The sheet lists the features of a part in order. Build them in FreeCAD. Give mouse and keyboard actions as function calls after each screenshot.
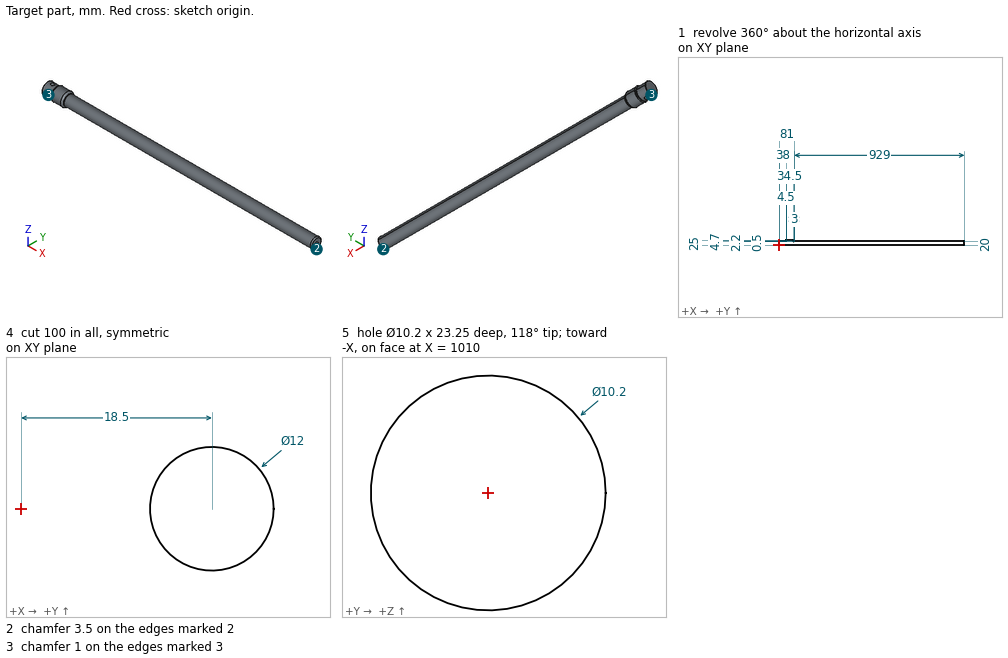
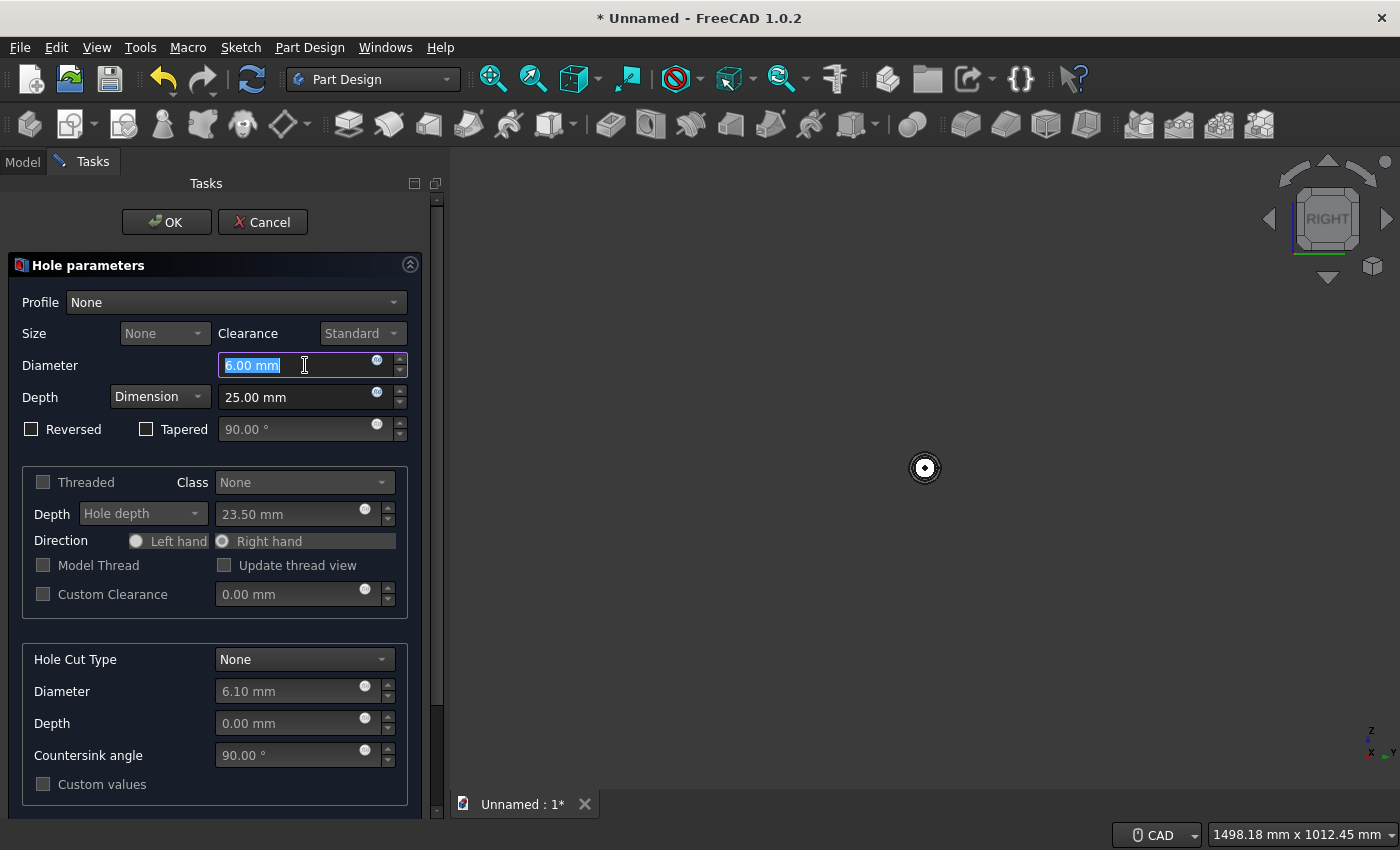
text(10.2)
key(Tab)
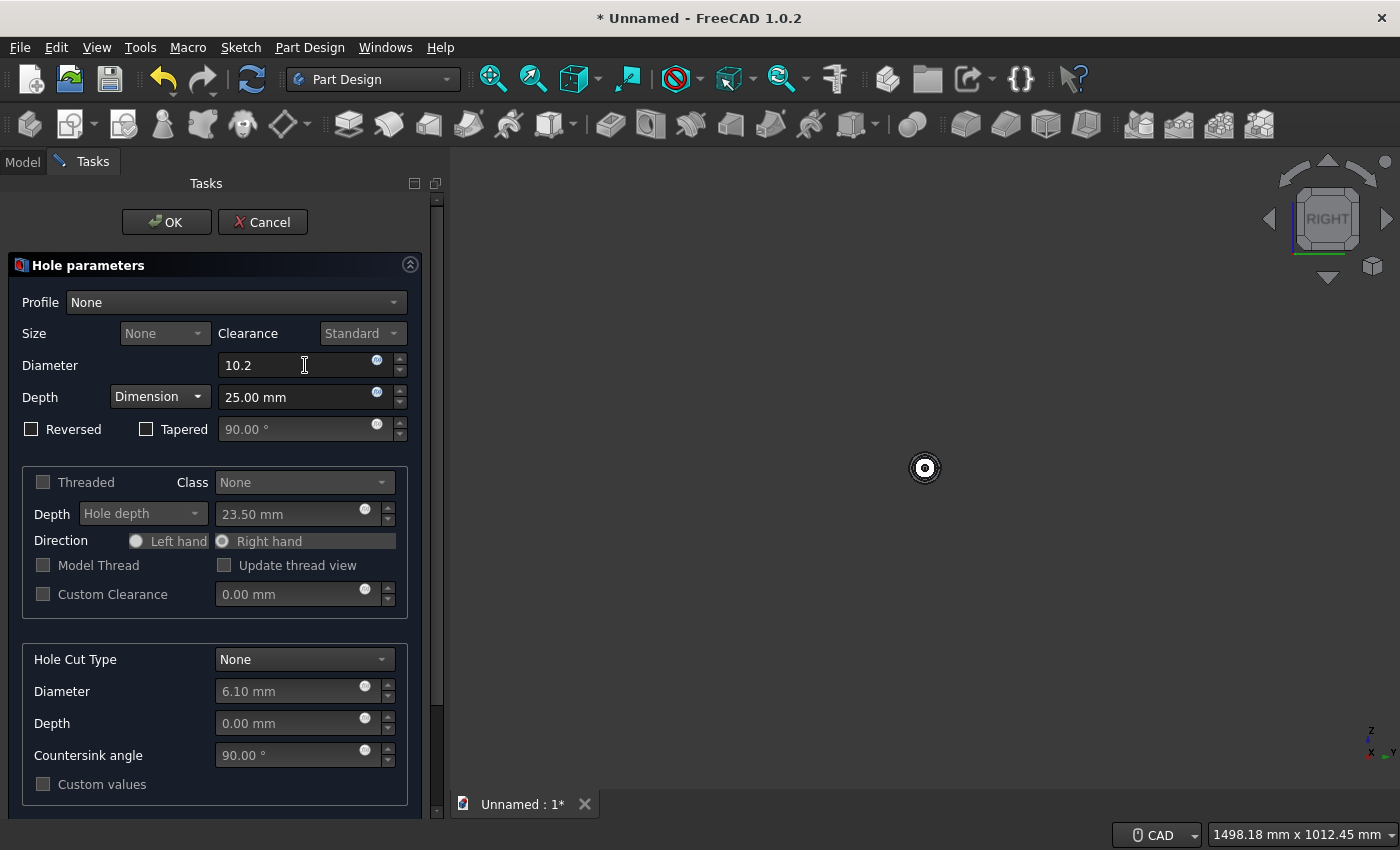
triple_click(305, 397)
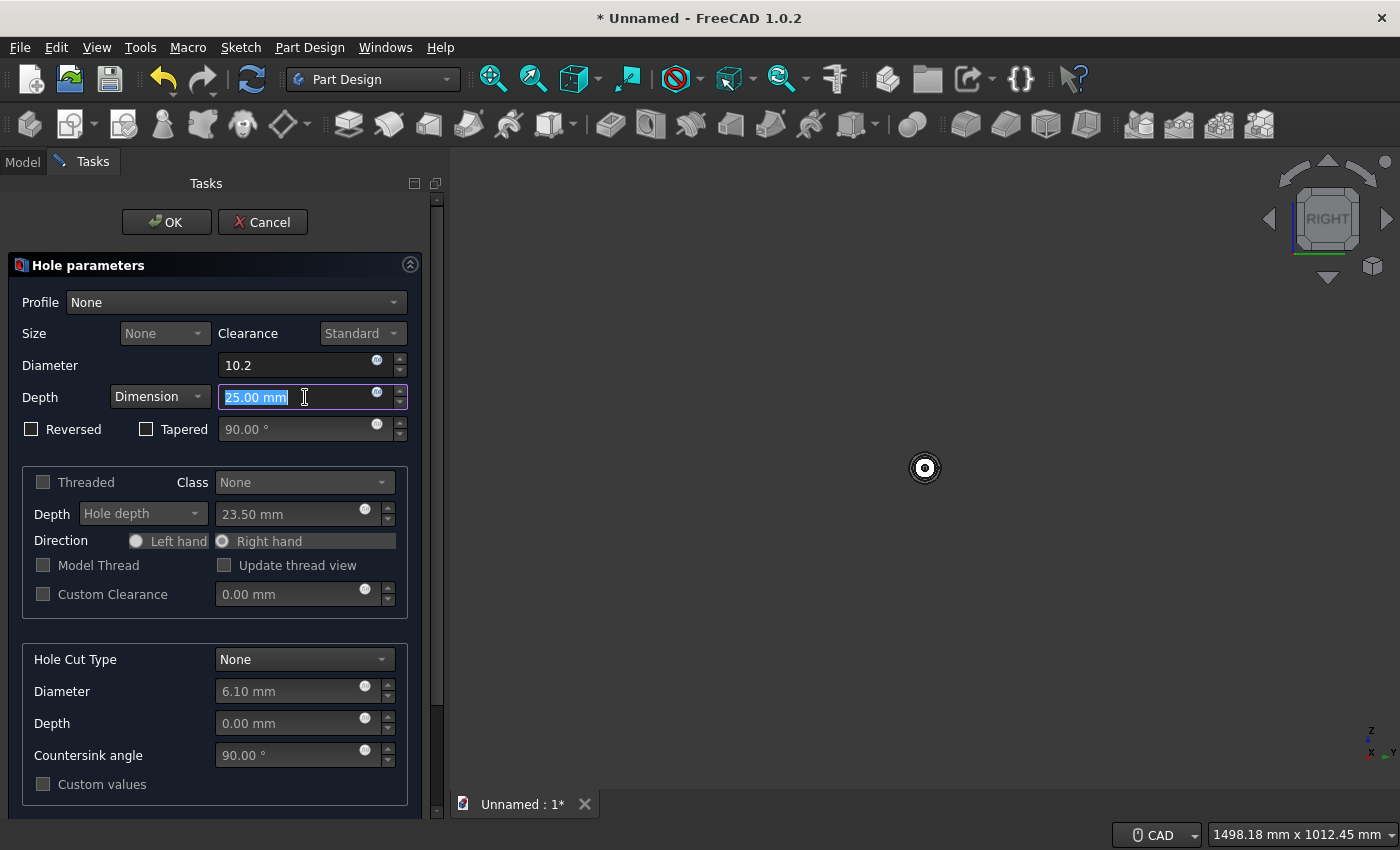
text(23.25)
key(Tab)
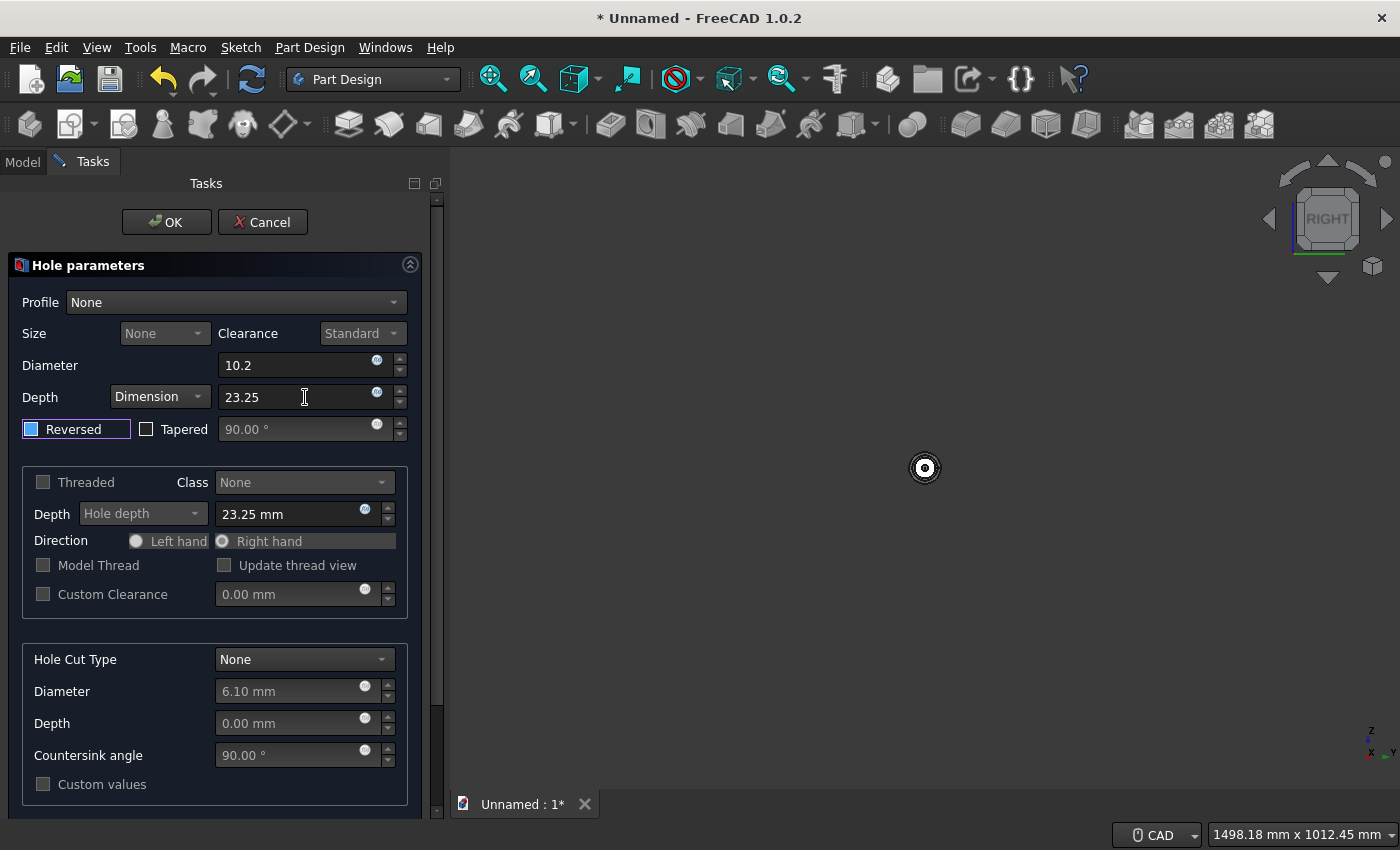
click(167, 222)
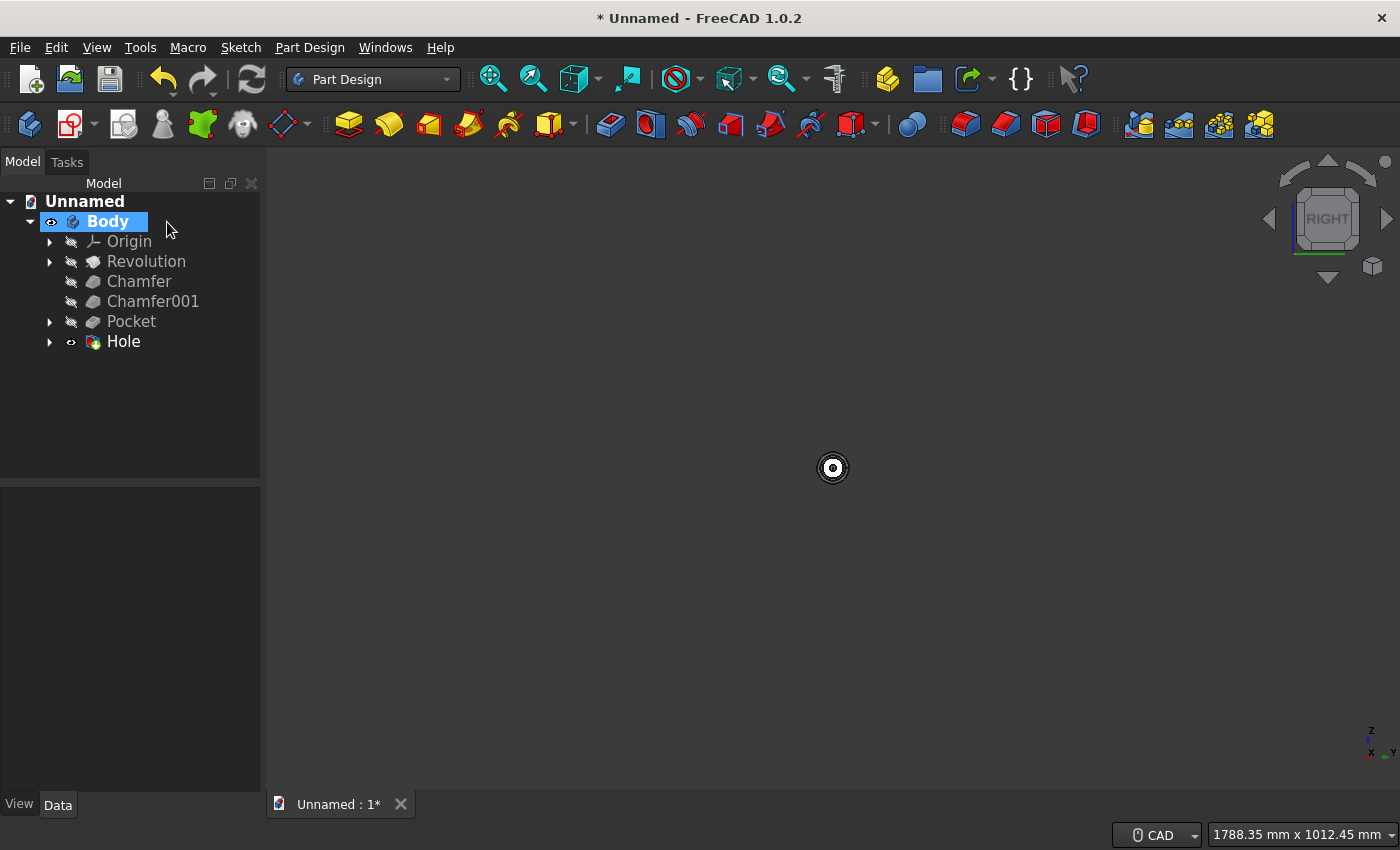
key(0)